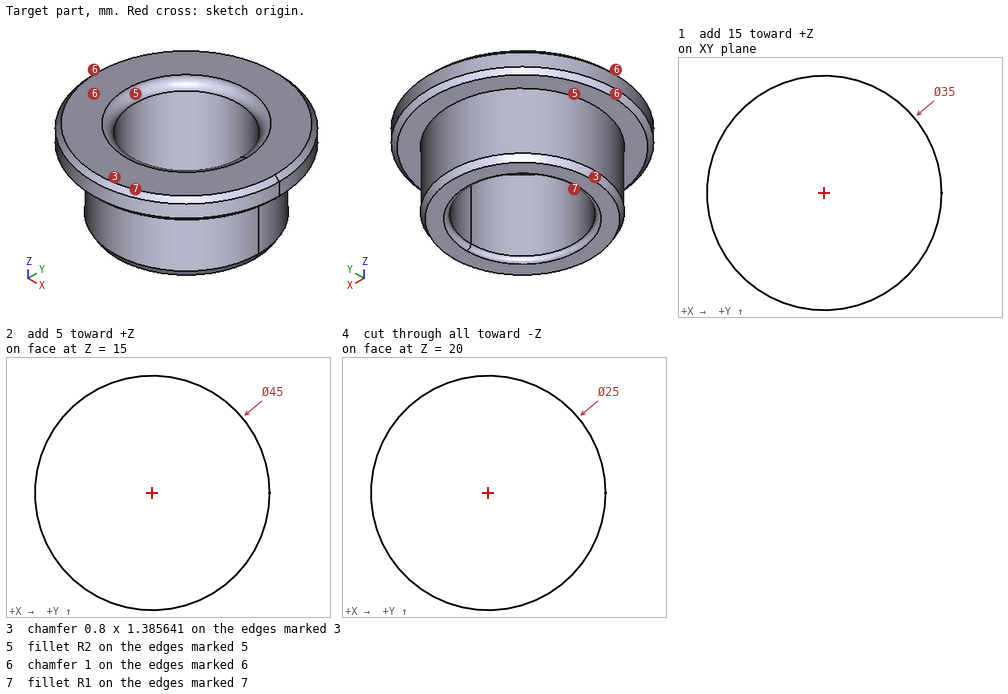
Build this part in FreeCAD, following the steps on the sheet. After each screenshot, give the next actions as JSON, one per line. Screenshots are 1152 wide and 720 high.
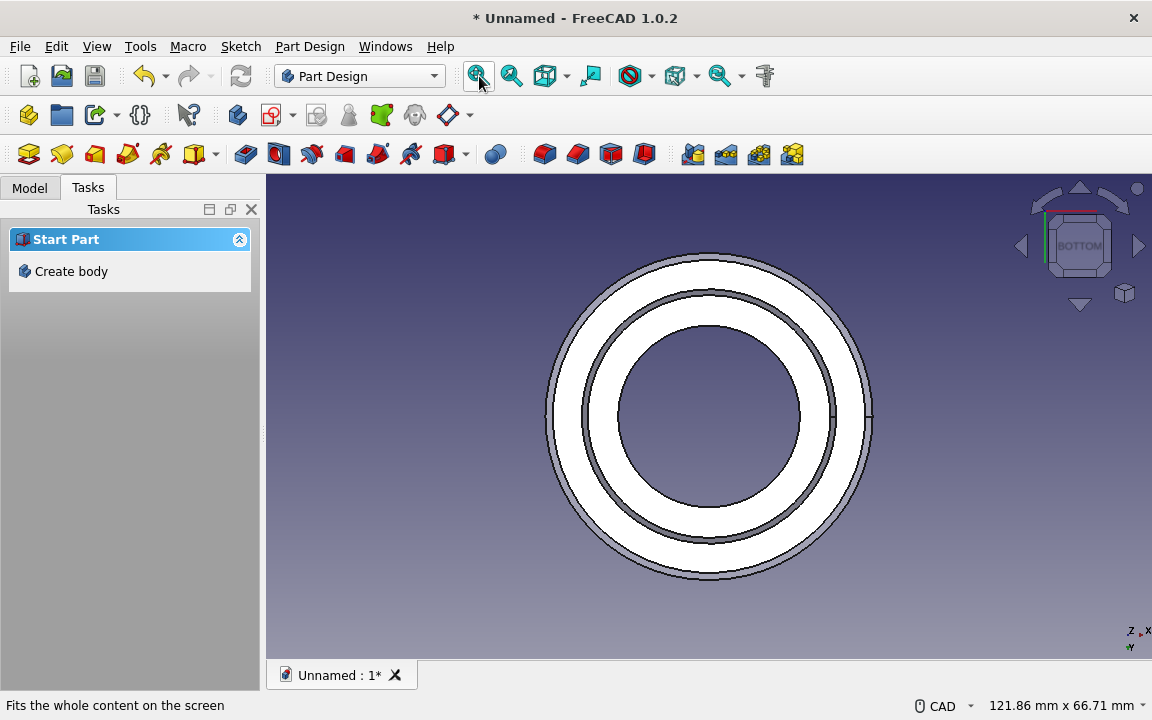
{"action": "left_click", "coordinate": [618, 415]}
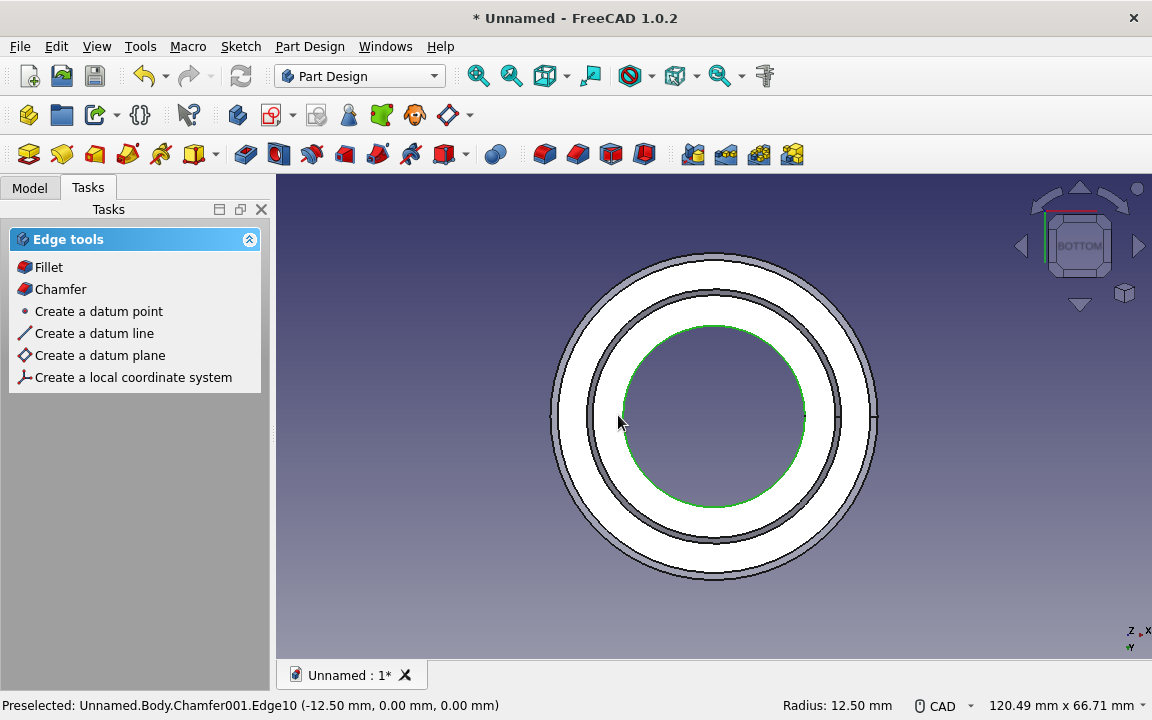
{"action": "left_click", "coordinate": [545, 154]}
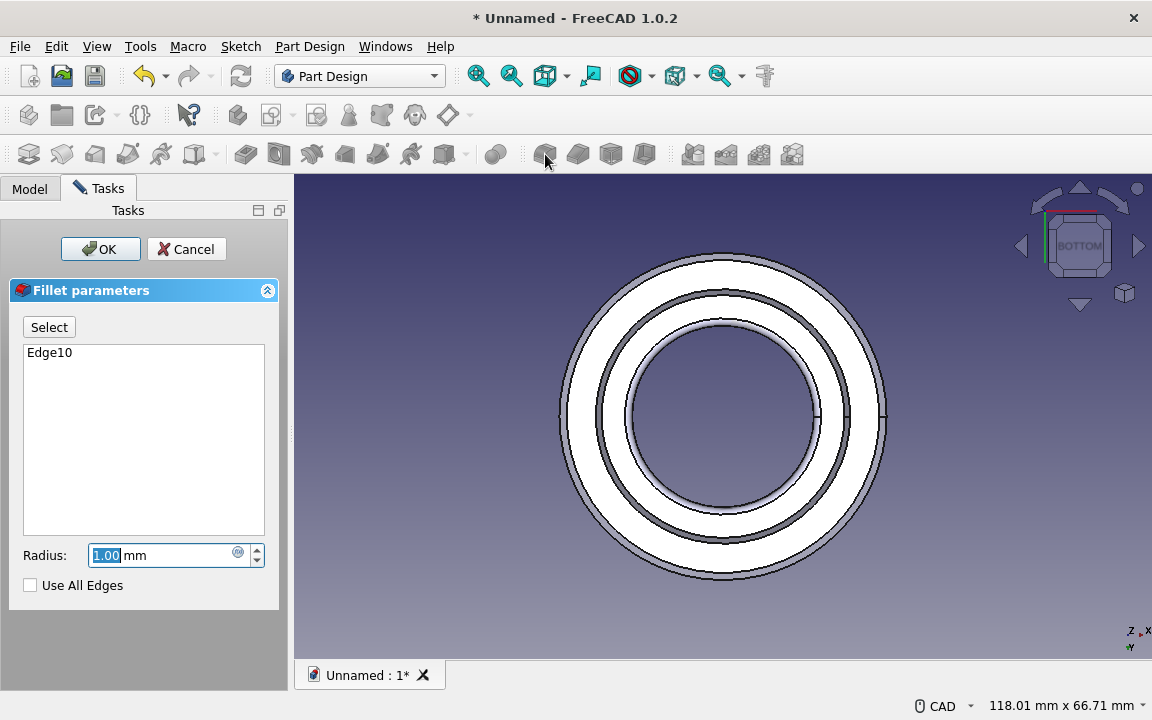
{"action": "type", "text": "1"}
{"action": "key", "text": "Tab"}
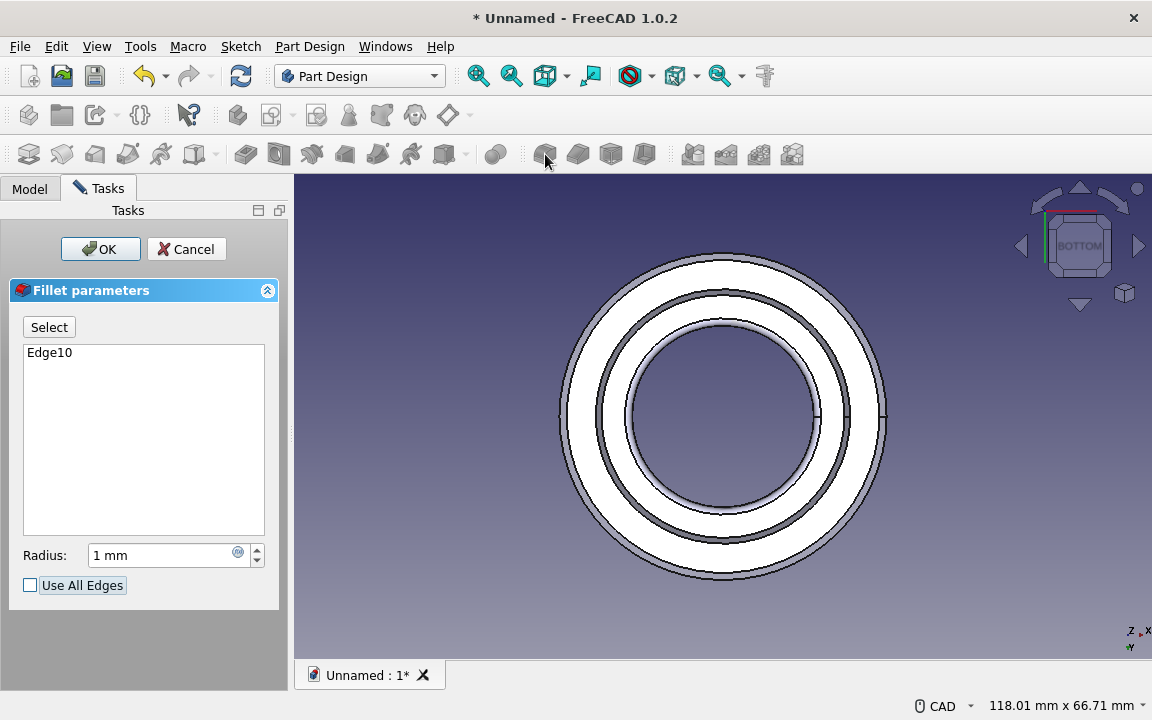
{"action": "left_click", "coordinate": [101, 249]}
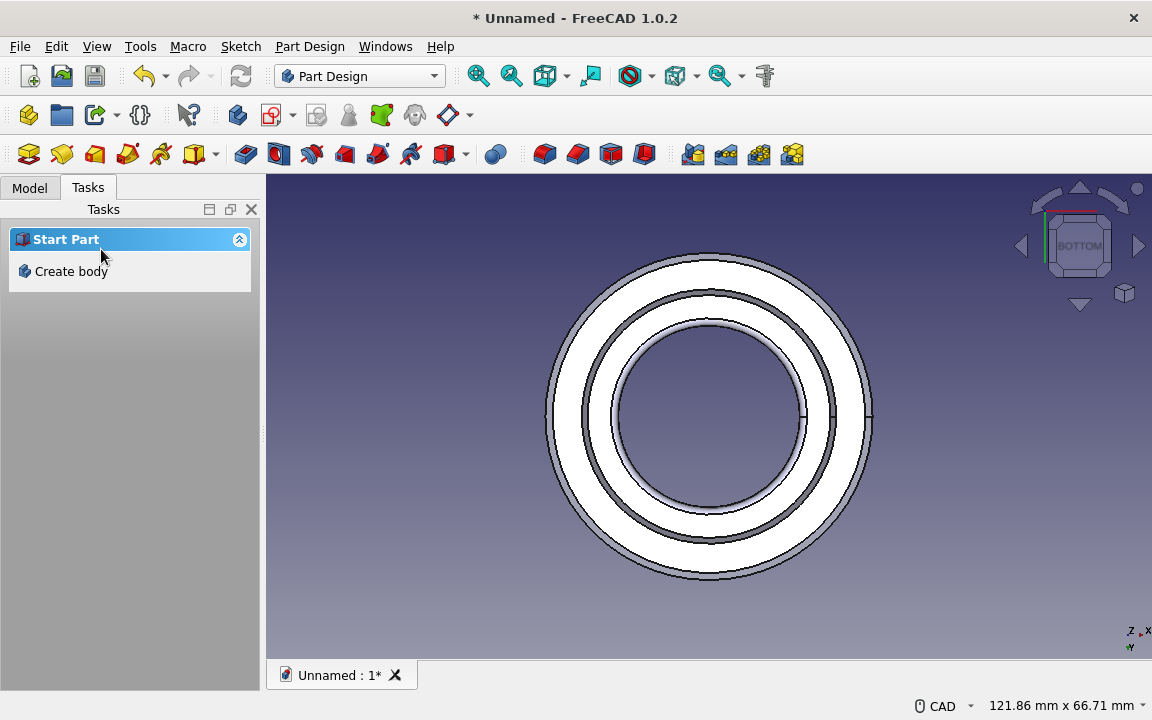
{"action": "key", "text": "0"}